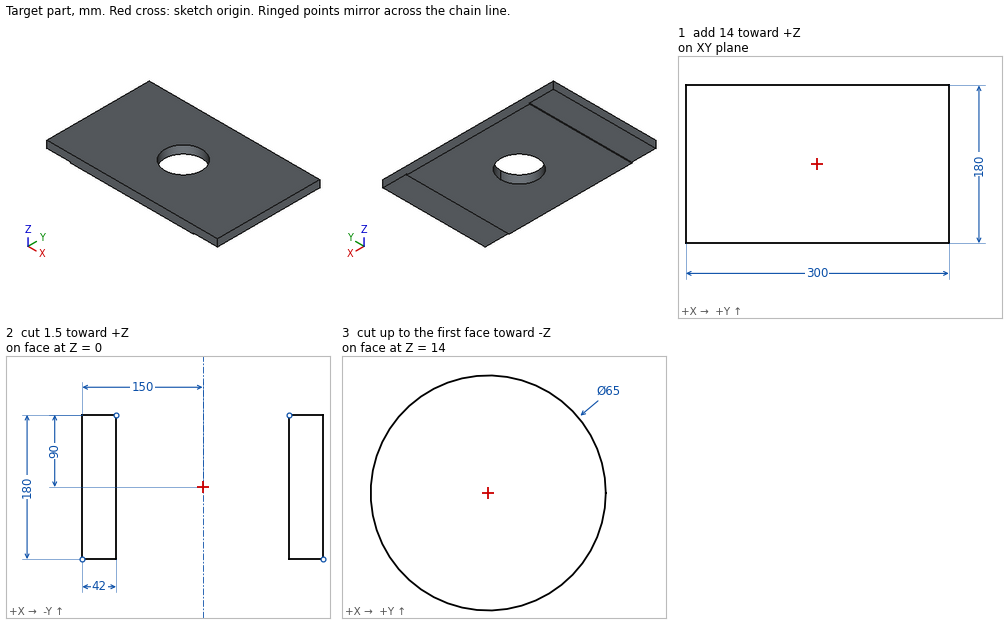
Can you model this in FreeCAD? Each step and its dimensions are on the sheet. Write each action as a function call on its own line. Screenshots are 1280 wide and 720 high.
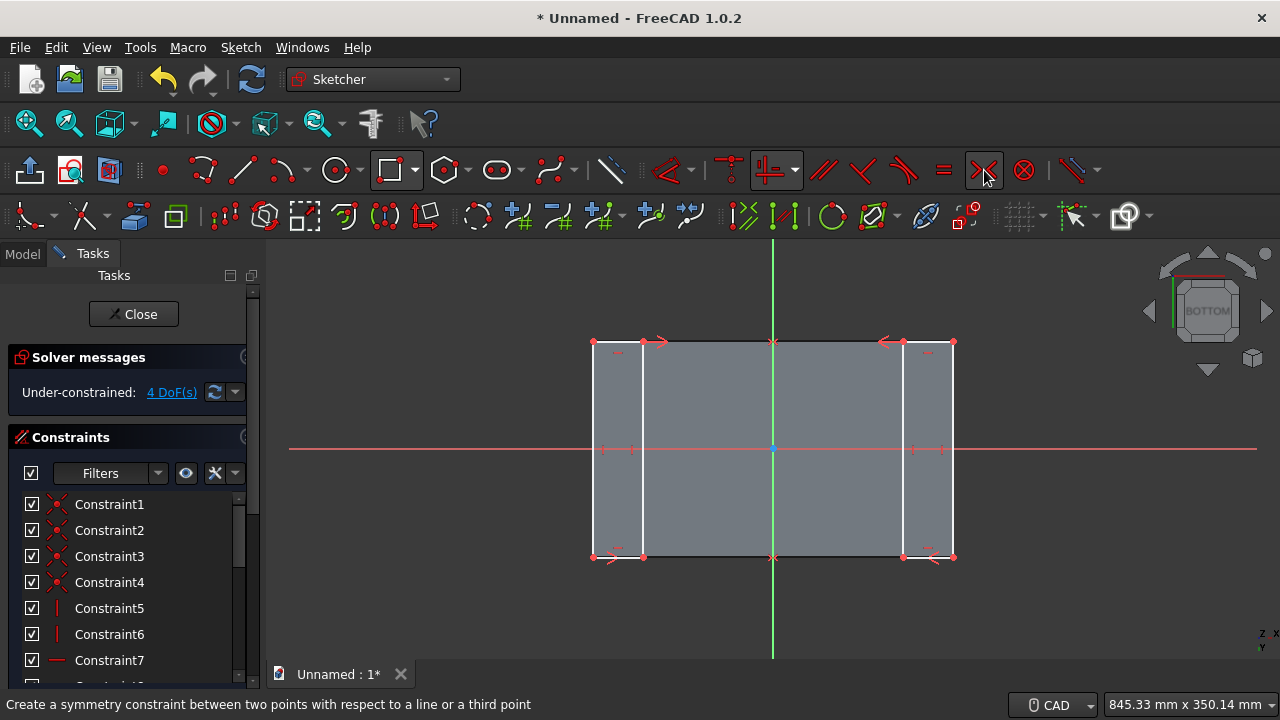
click(666, 170)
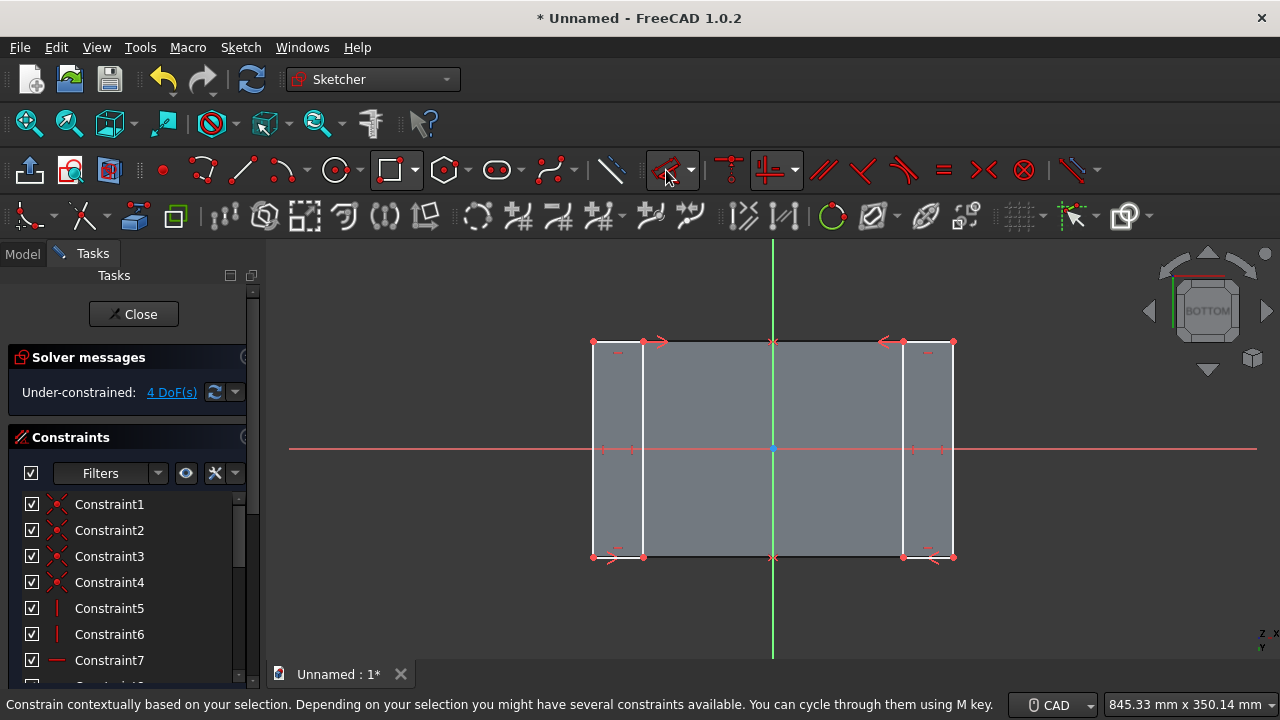
click(608, 558)
click(618, 592)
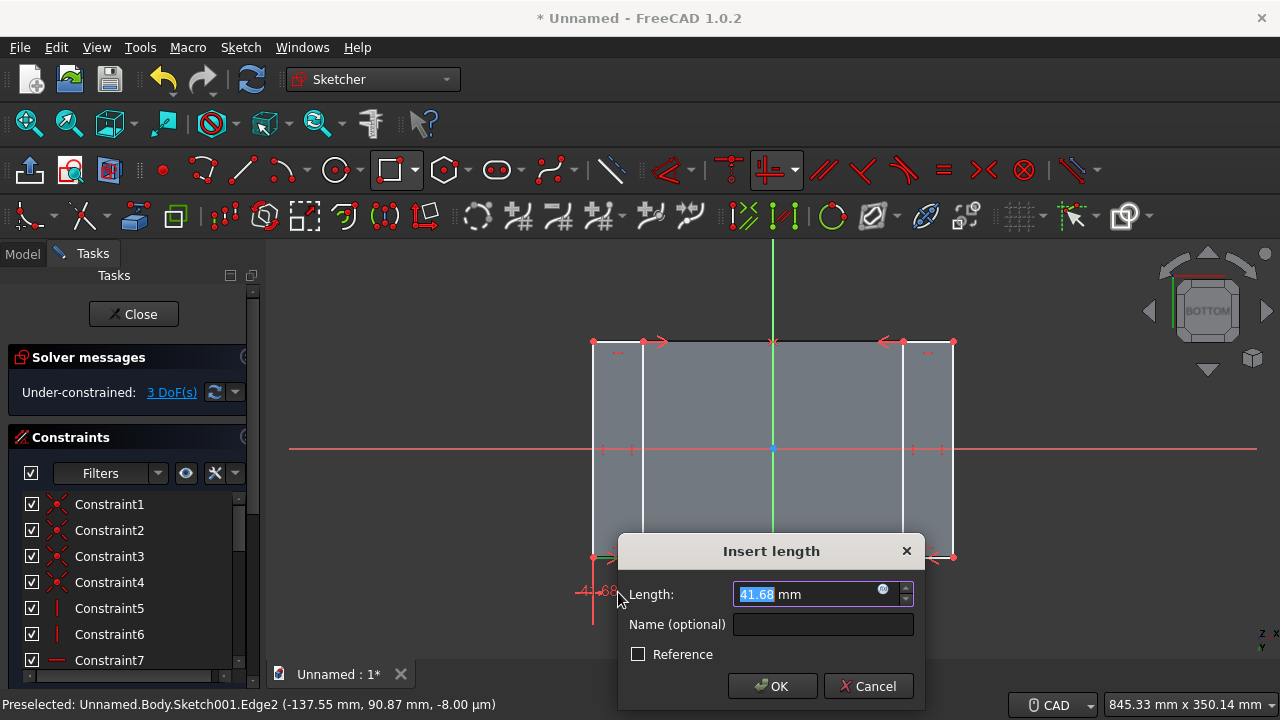
text(42)
key(Return)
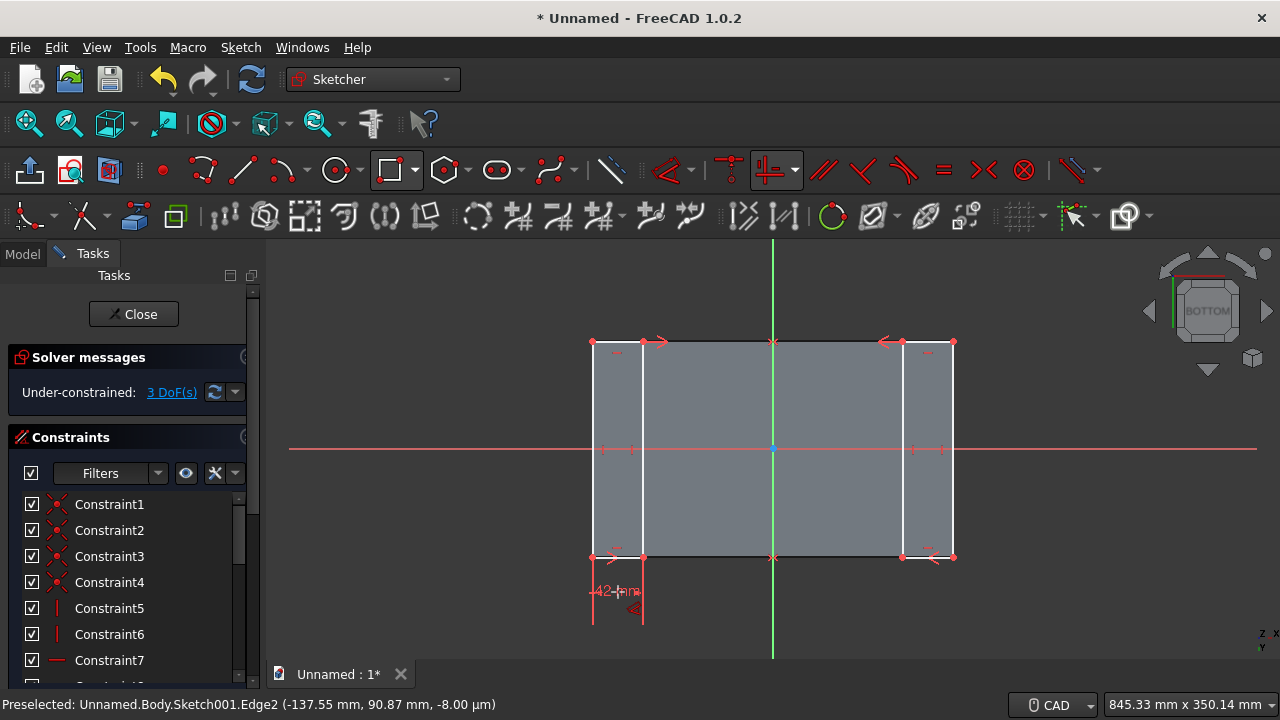
click(593, 407)
click(559, 400)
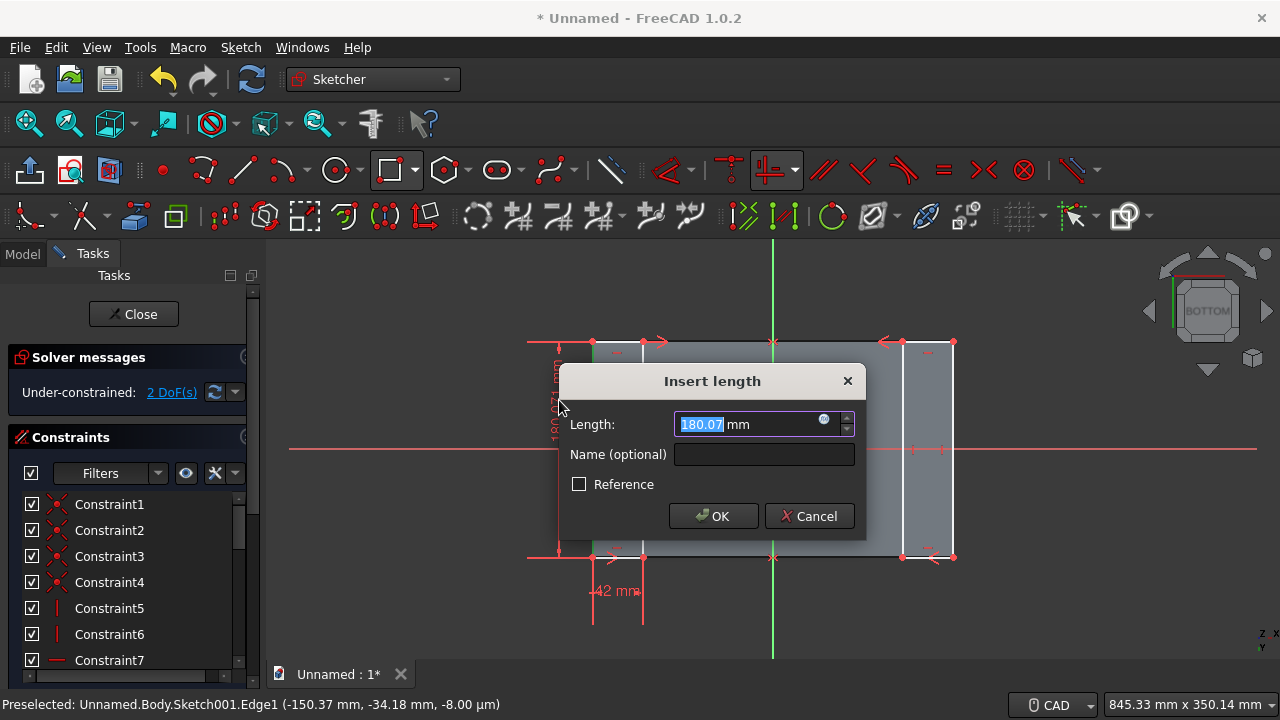
text(180)
key(Return)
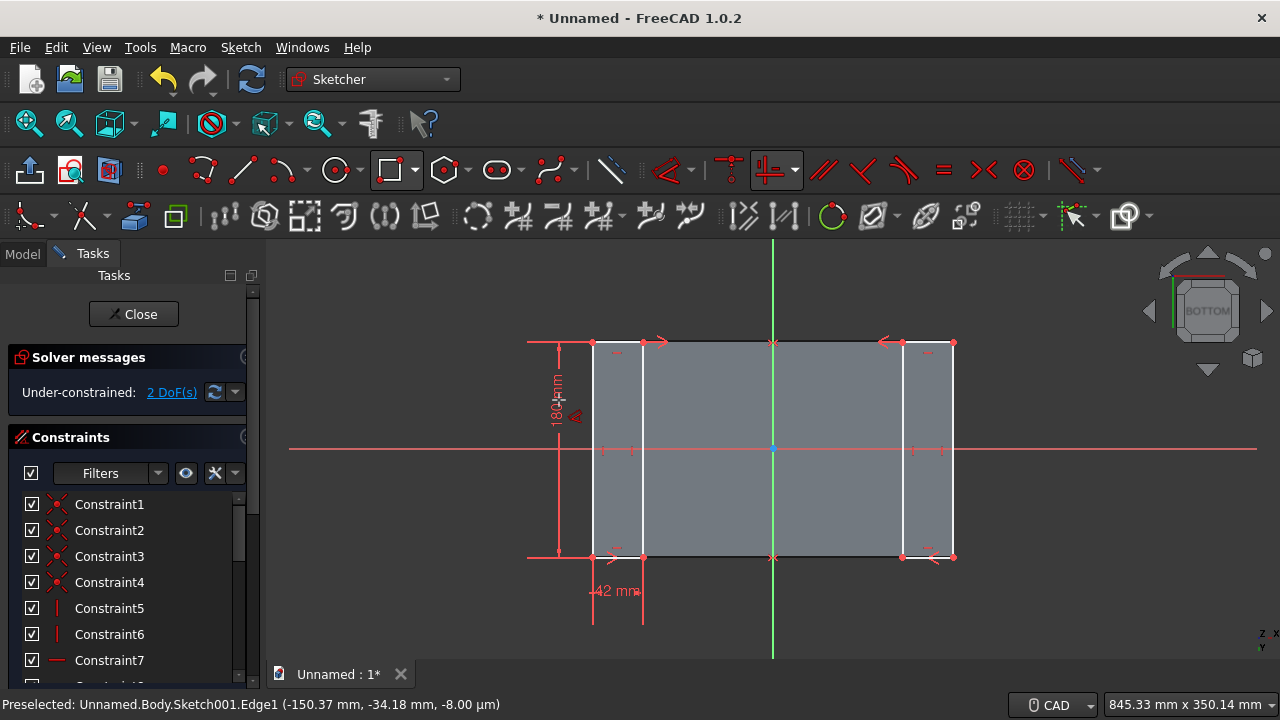
click(593, 342)
click(559, 371)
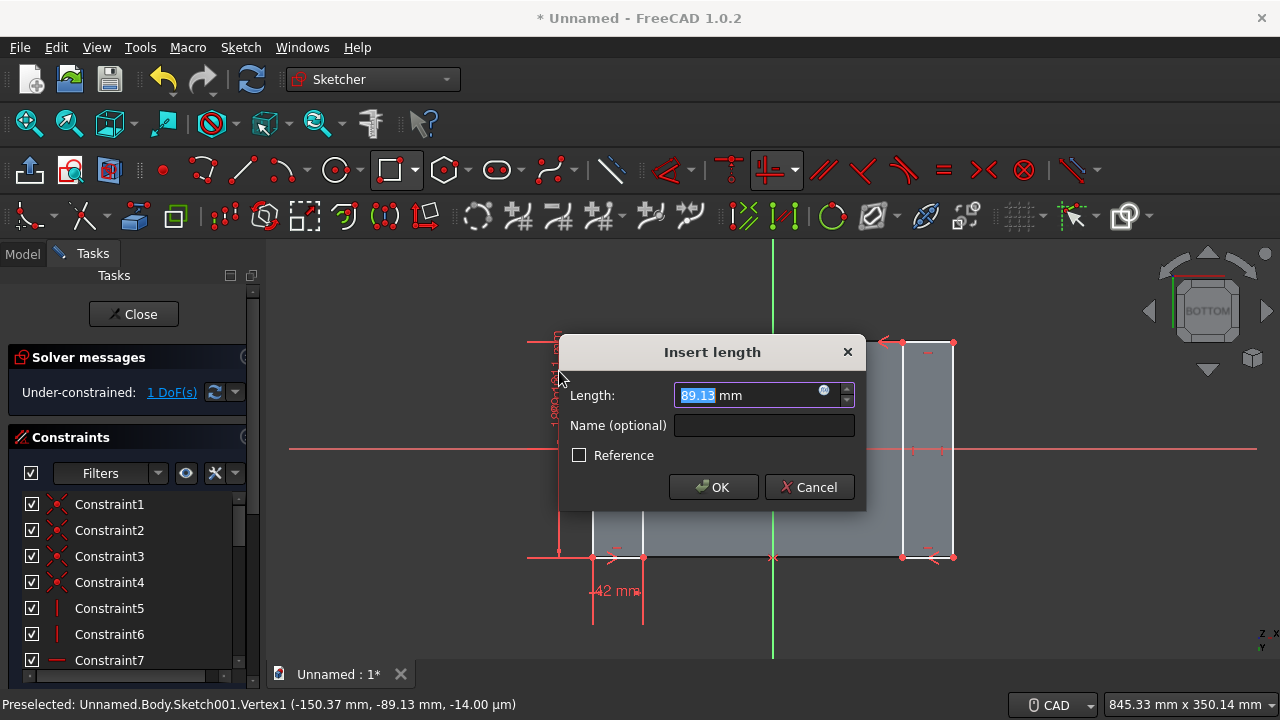
text(90)
key(Return)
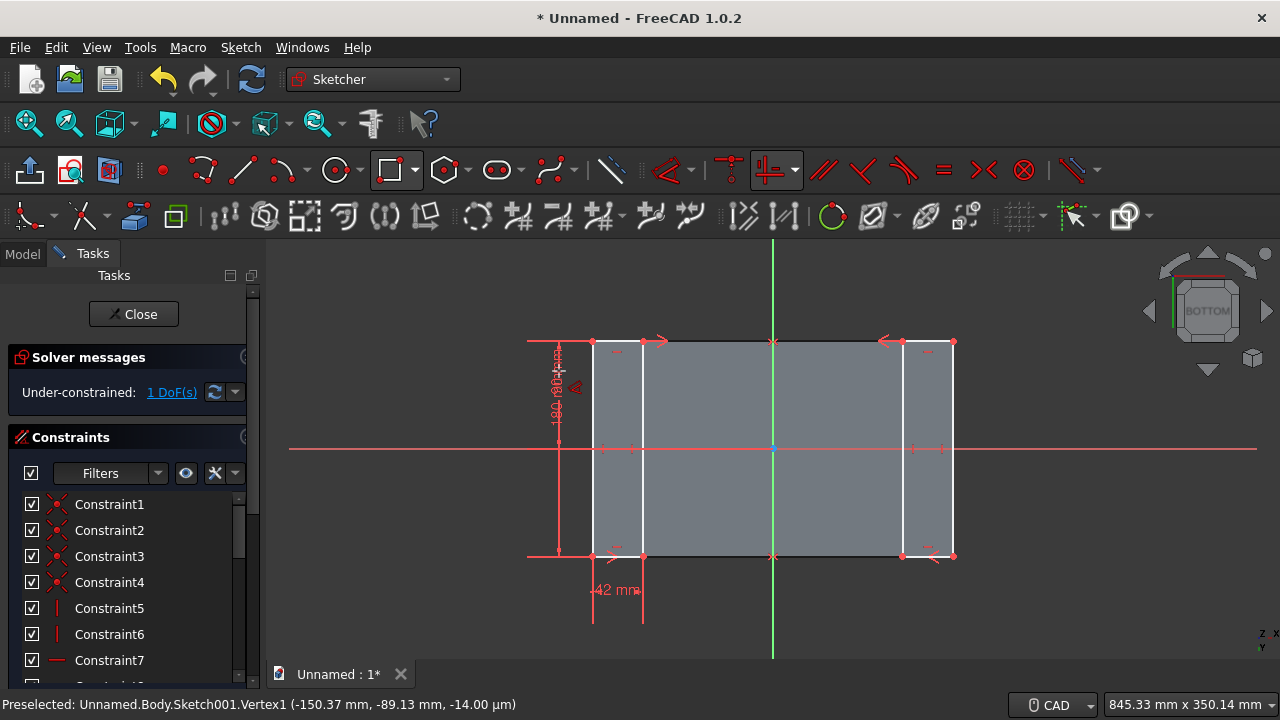
click(593, 341)
click(683, 307)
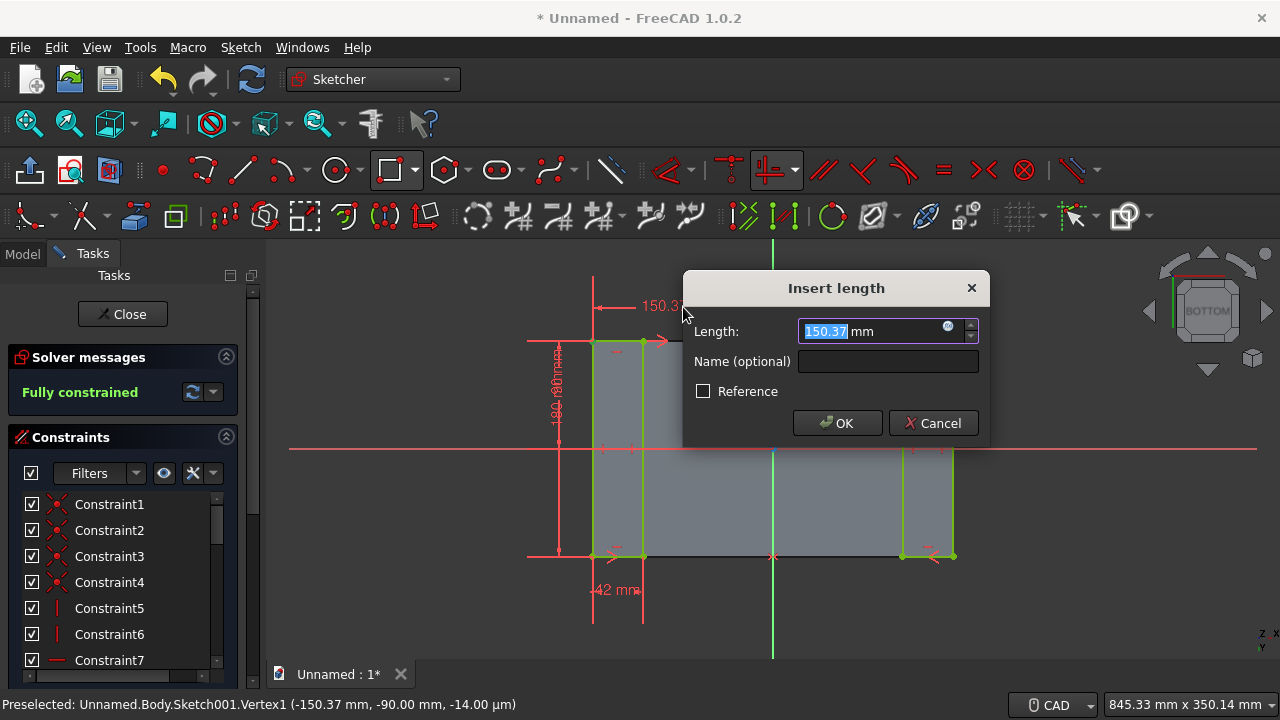
text(150)
key(Return)
key(Escape)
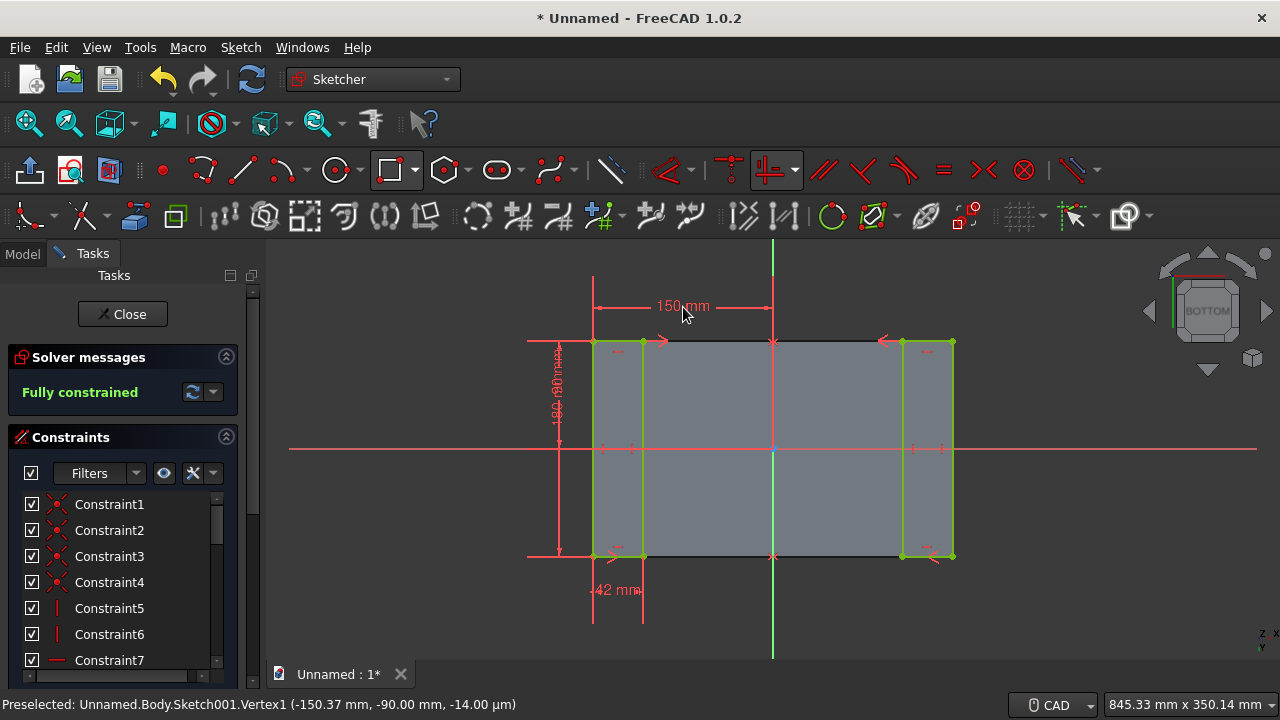
click(123, 314)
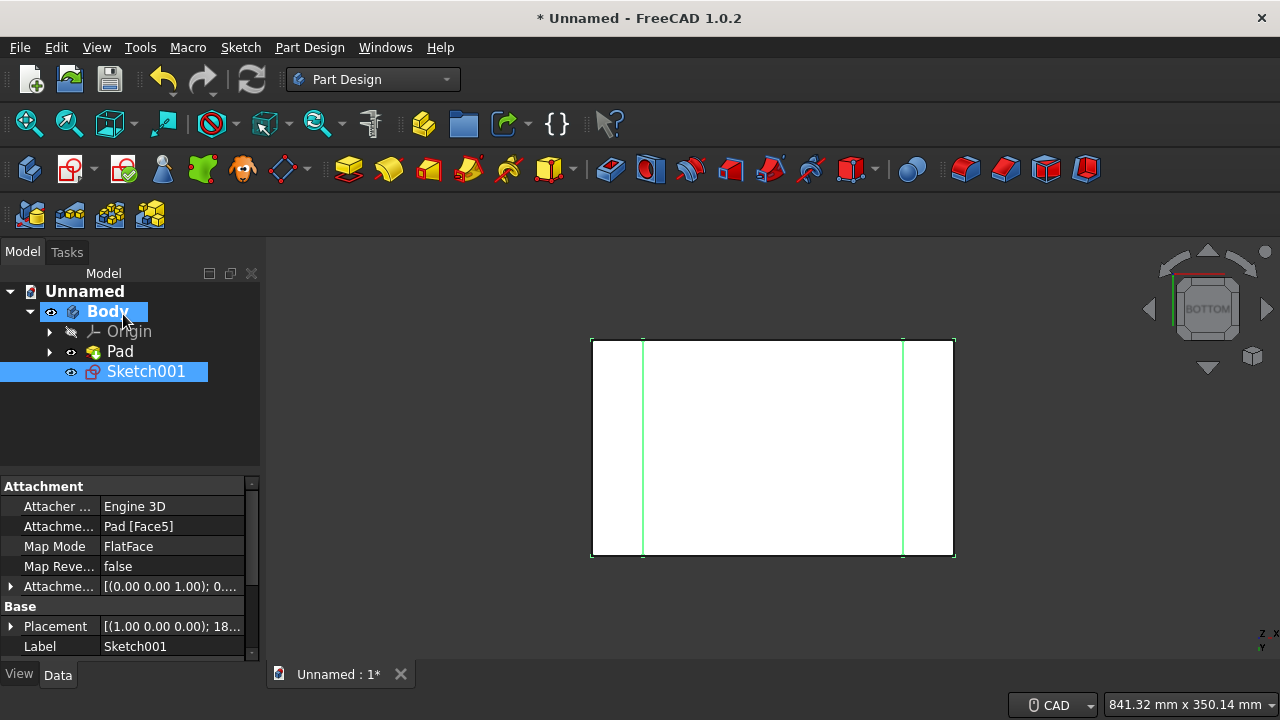
click(612, 170)